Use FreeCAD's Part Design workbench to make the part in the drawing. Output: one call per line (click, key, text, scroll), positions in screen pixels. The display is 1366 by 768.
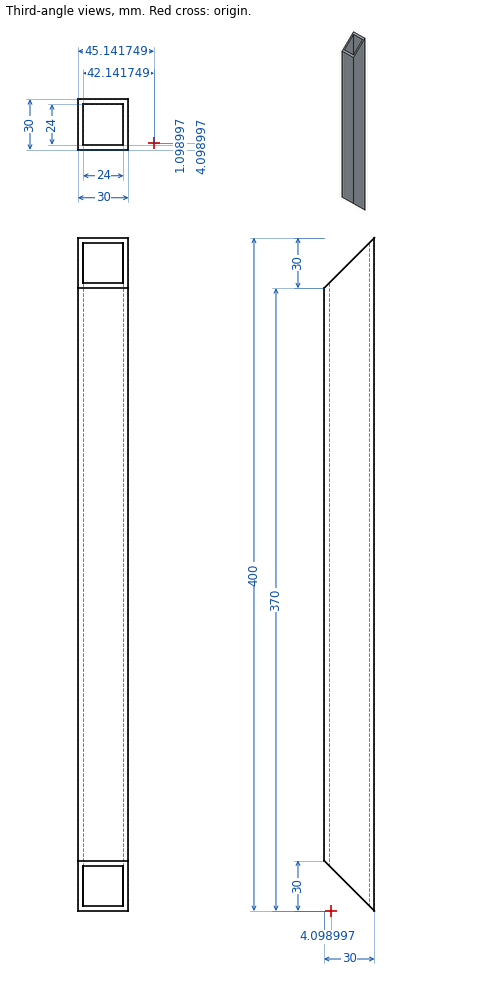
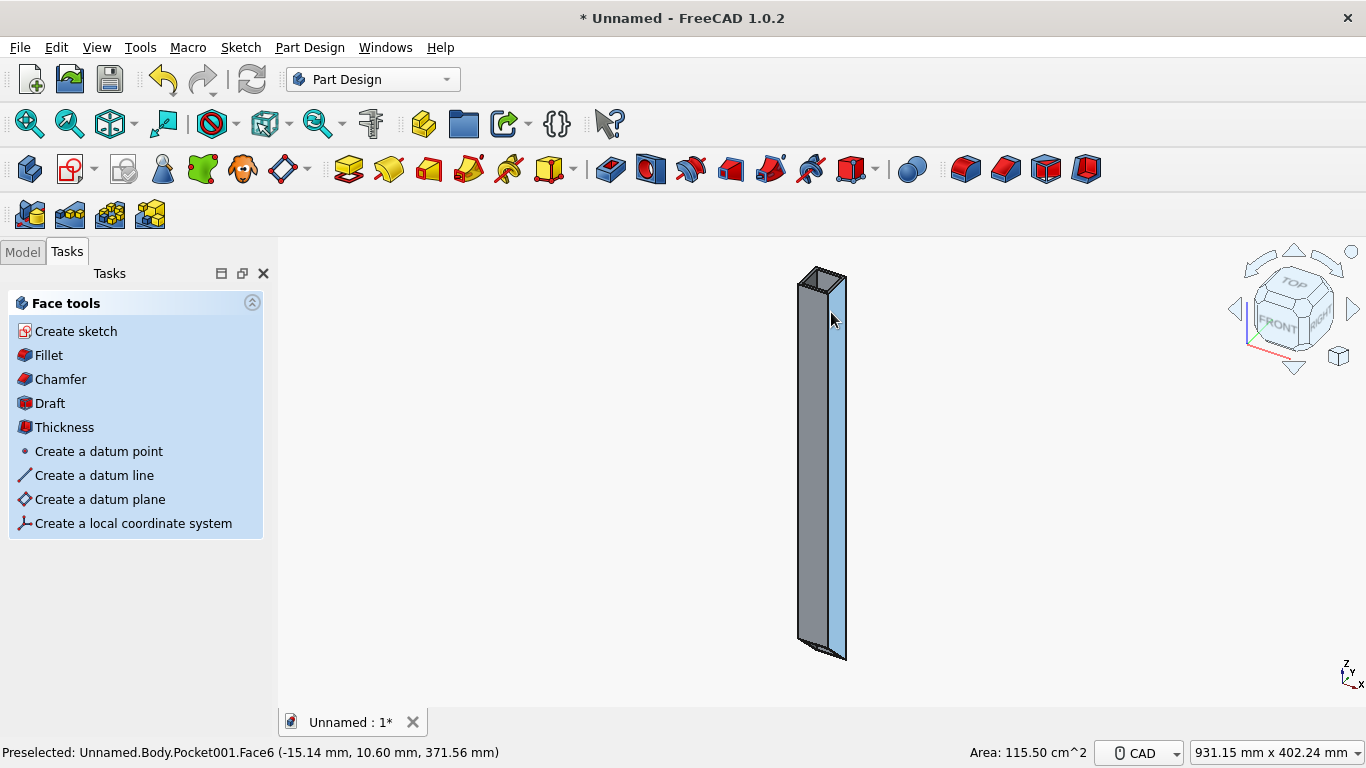
click(70, 170)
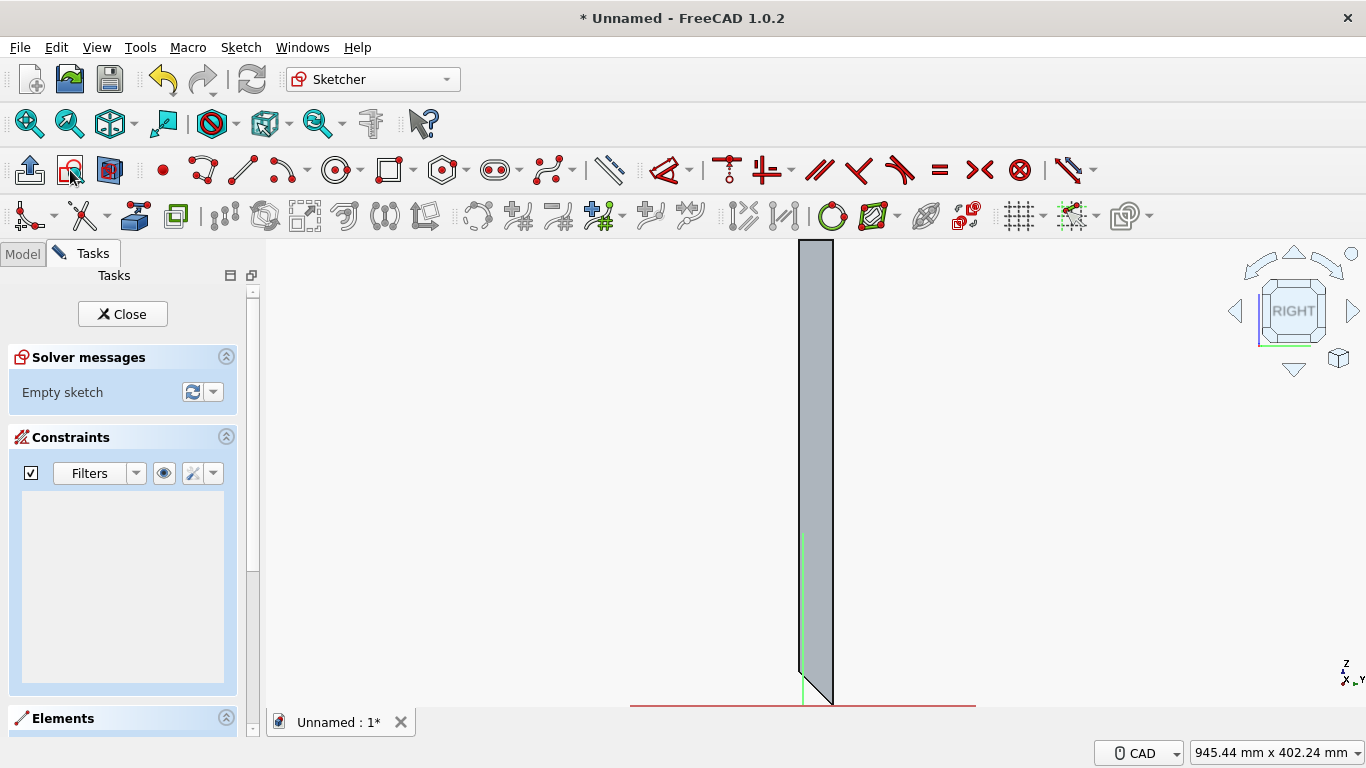
scroll(748, 473, down, 5)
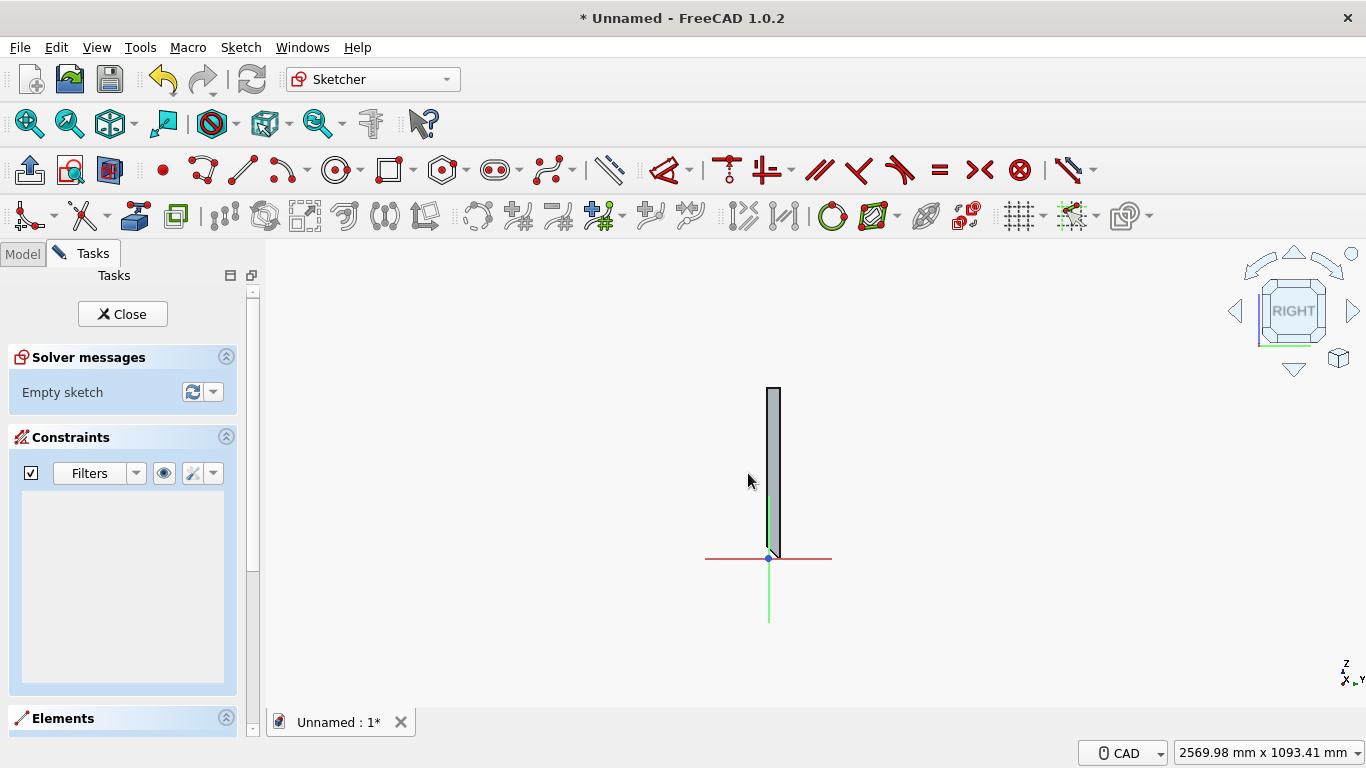
scroll(775, 390, up, 15)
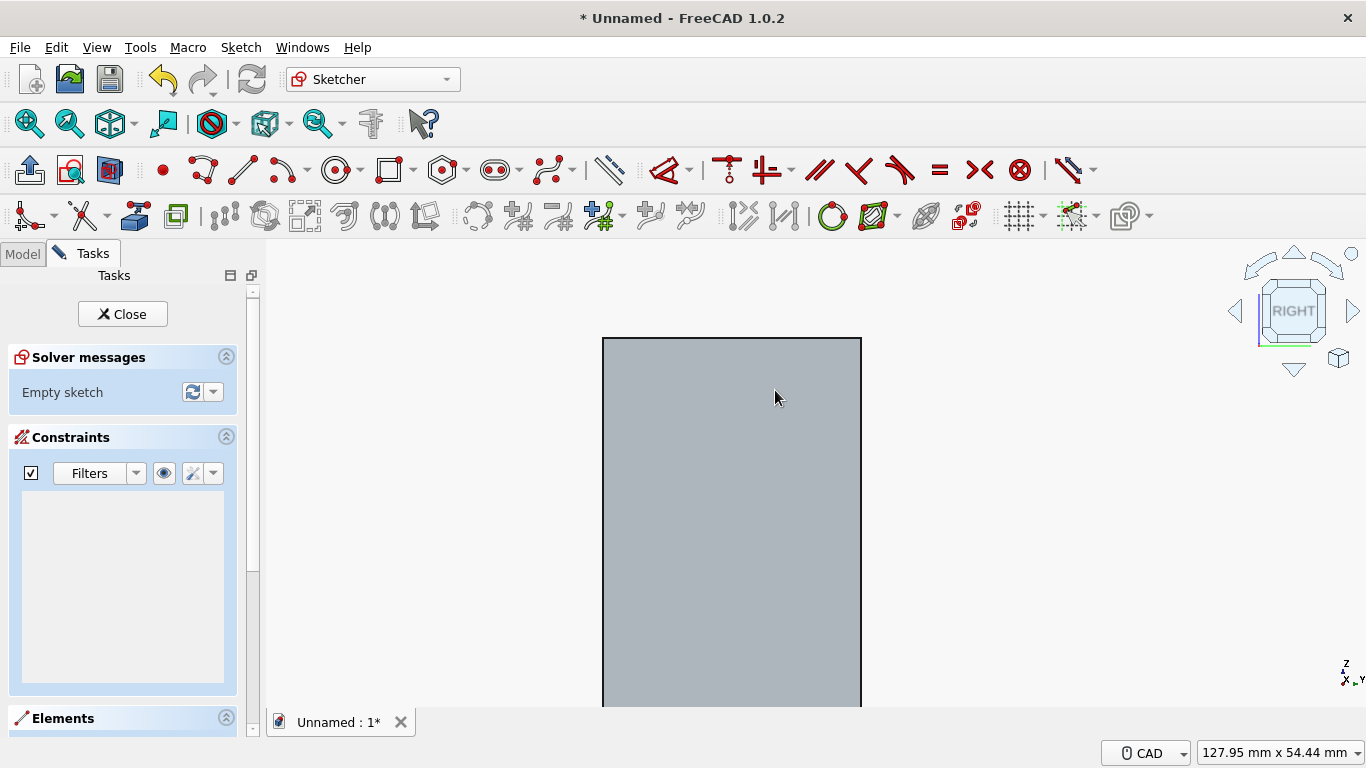
click(204, 170)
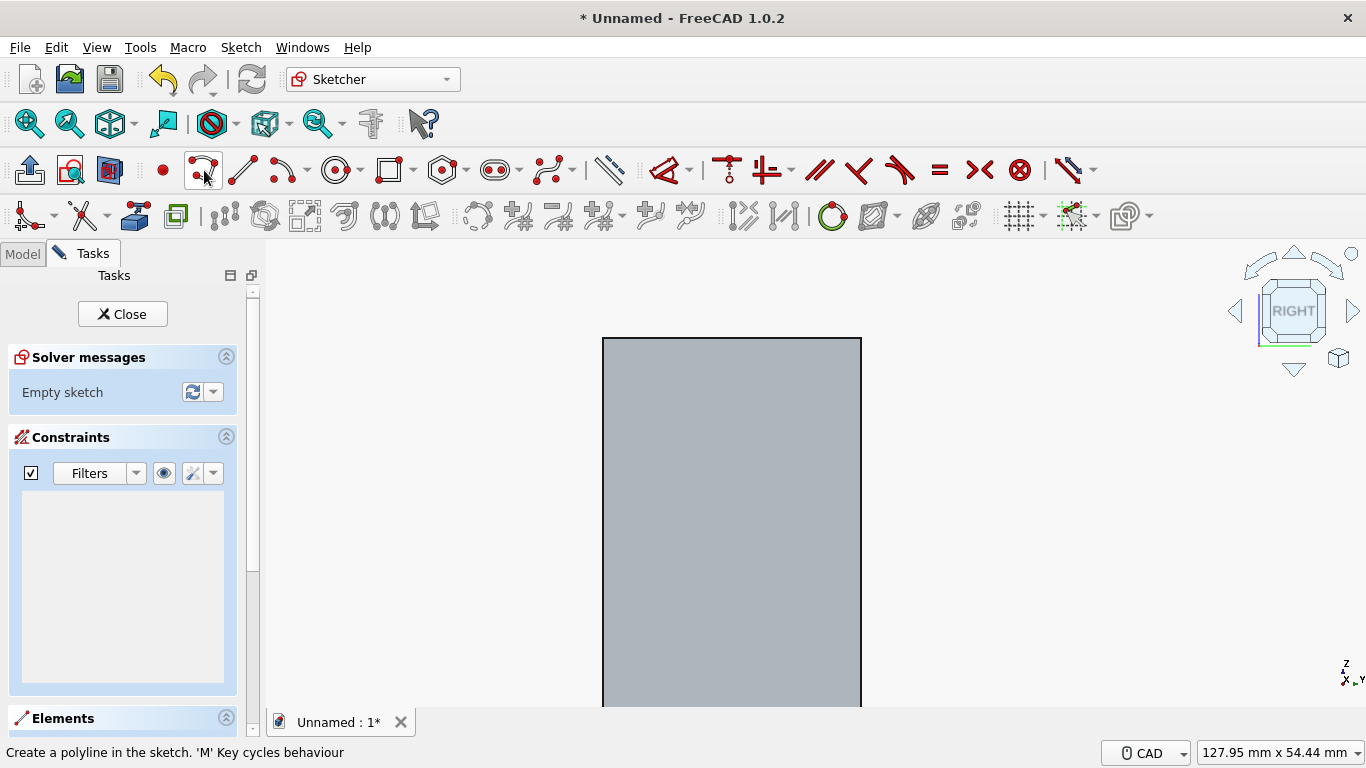
click(603, 596)
click(861, 338)
click(603, 338)
click(603, 597)
key(Escape)
key(Escape)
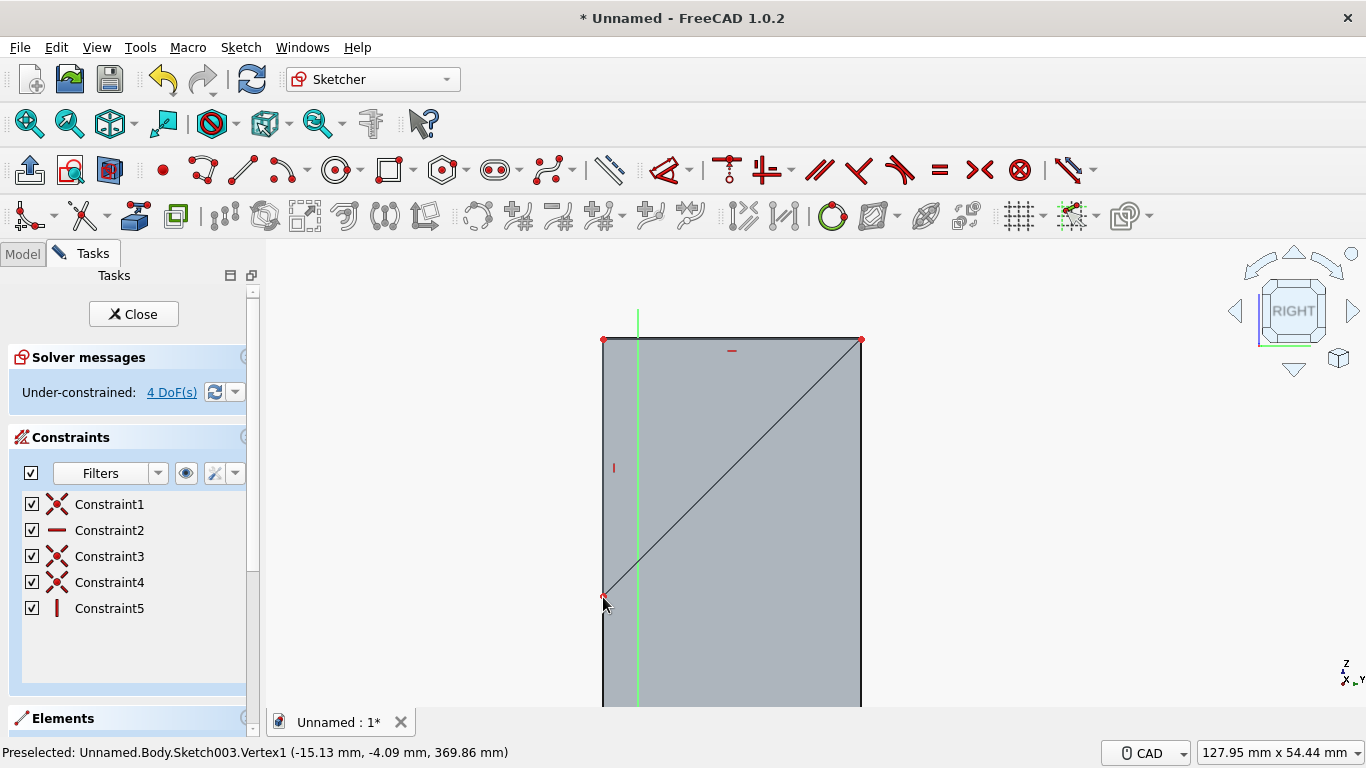
click(664, 170)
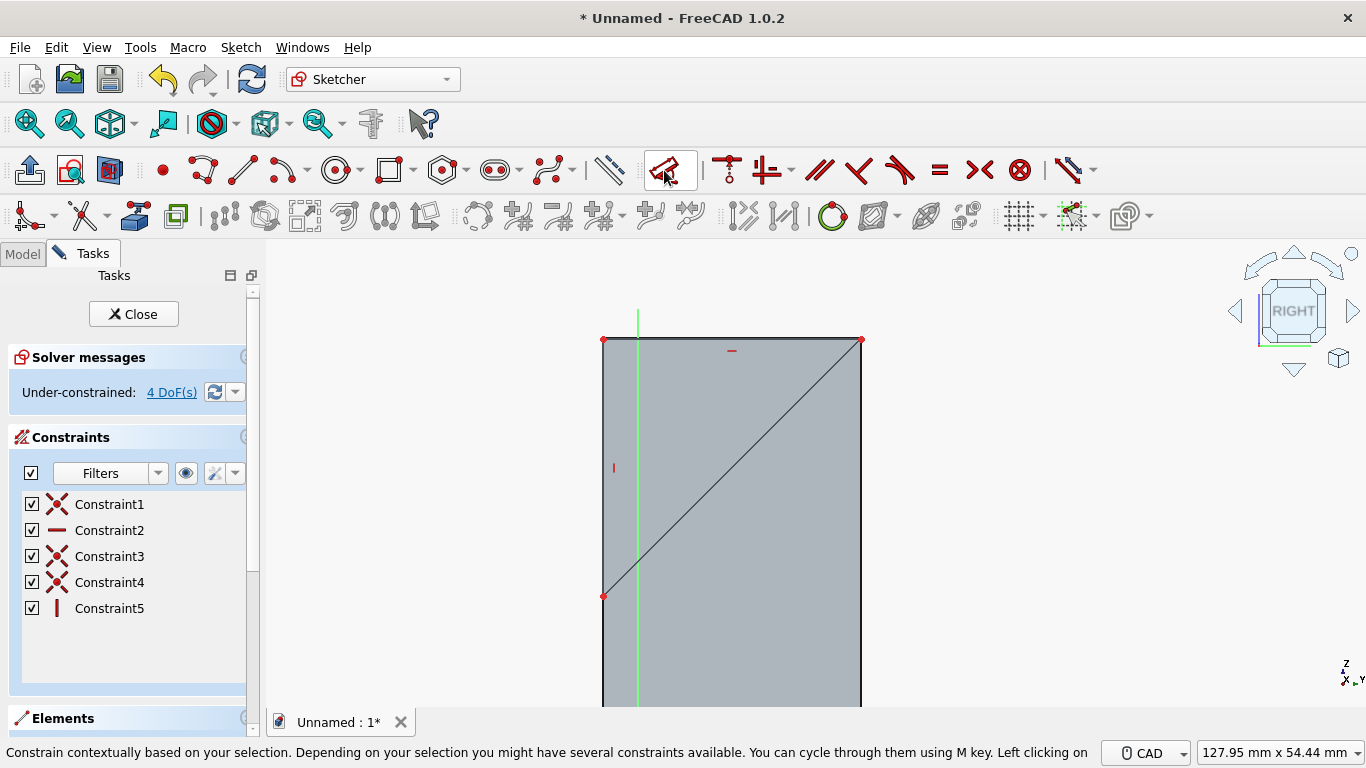
click(784, 339)
click(732, 305)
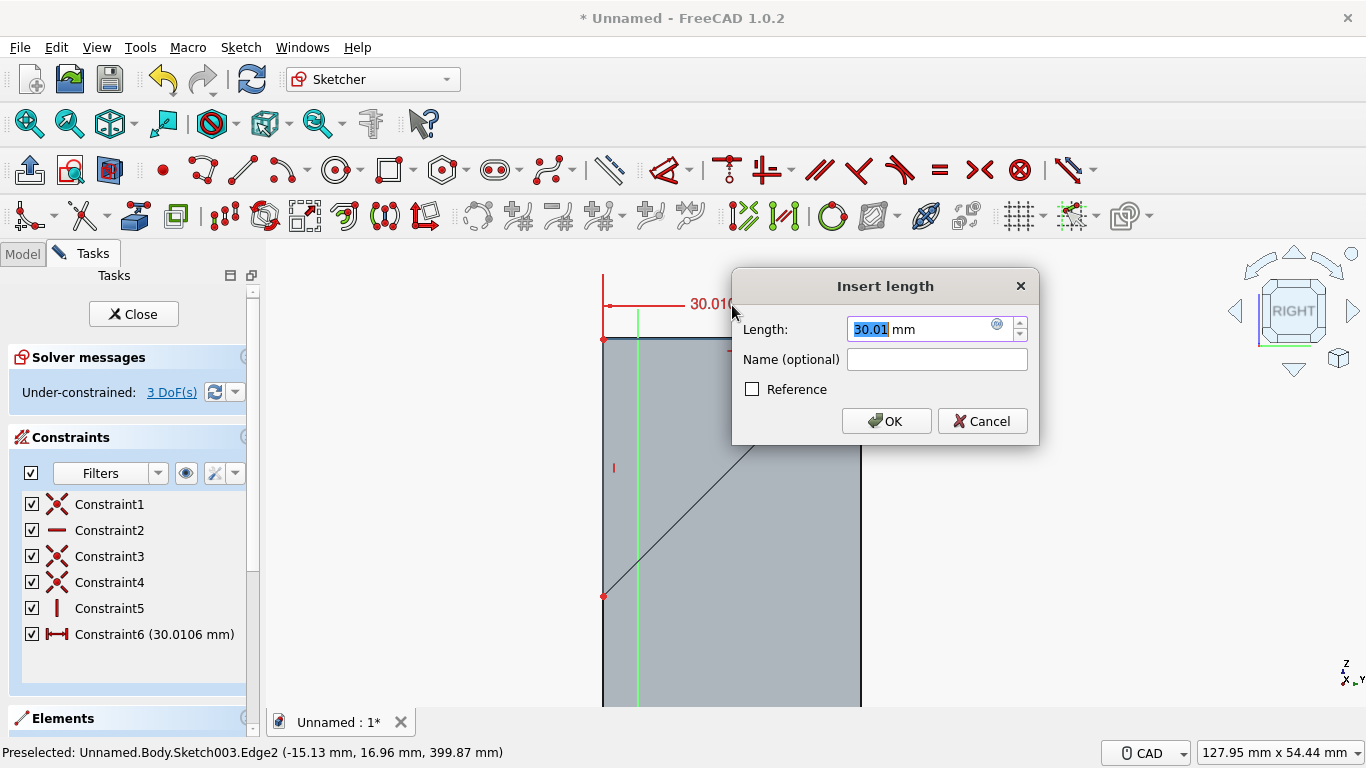
text(30)
key(Return)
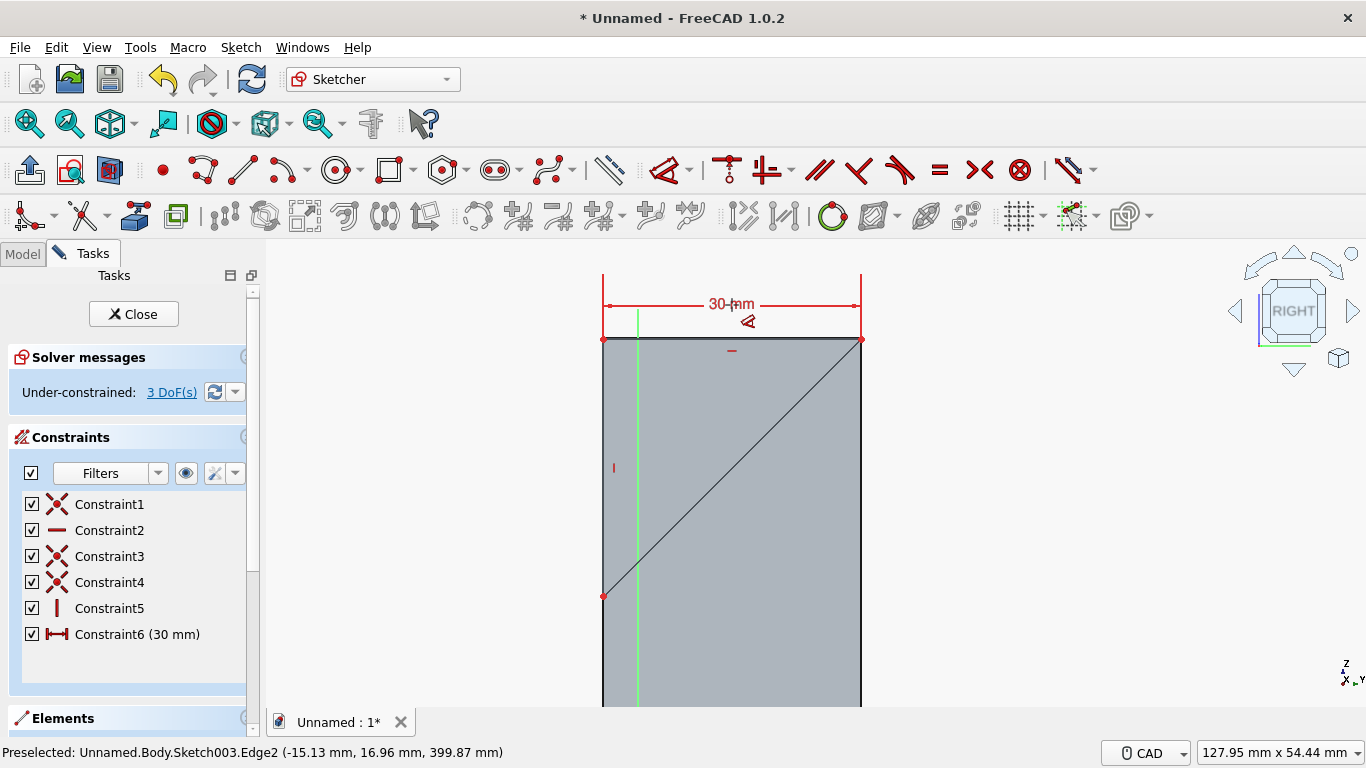
click(603, 416)
click(569, 468)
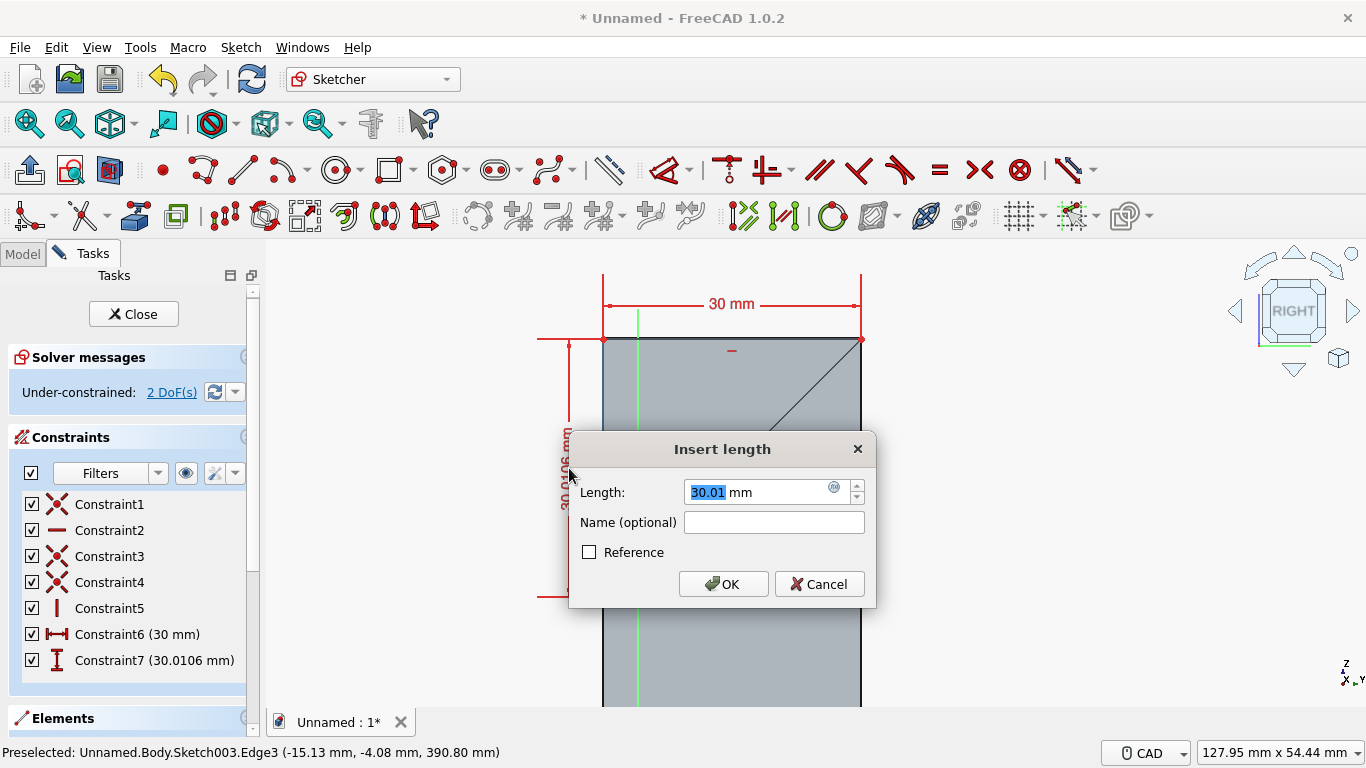
text(30)
key(Return)